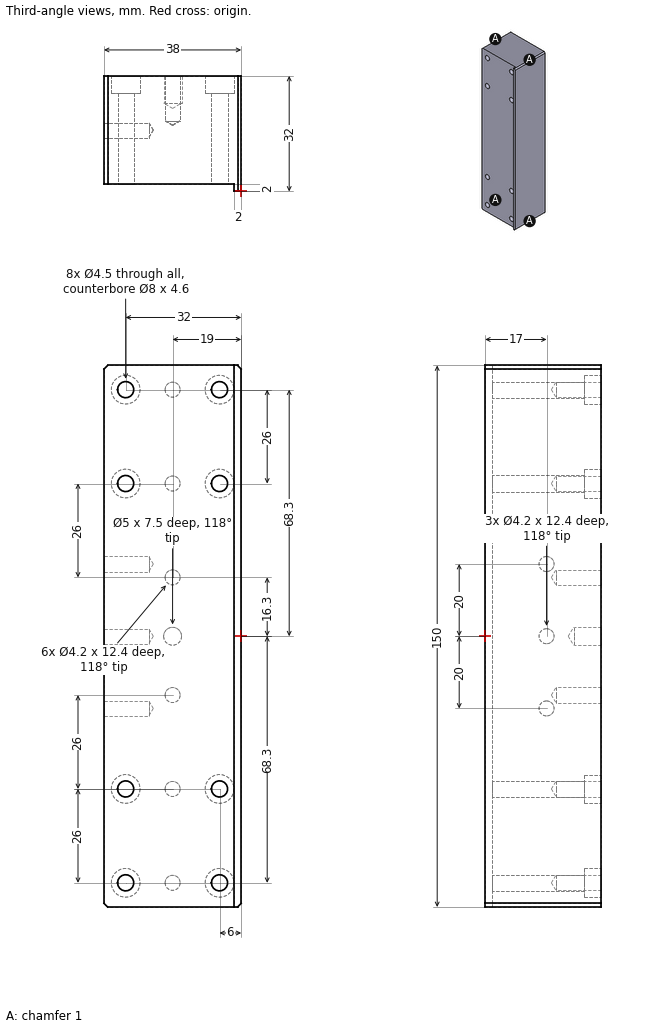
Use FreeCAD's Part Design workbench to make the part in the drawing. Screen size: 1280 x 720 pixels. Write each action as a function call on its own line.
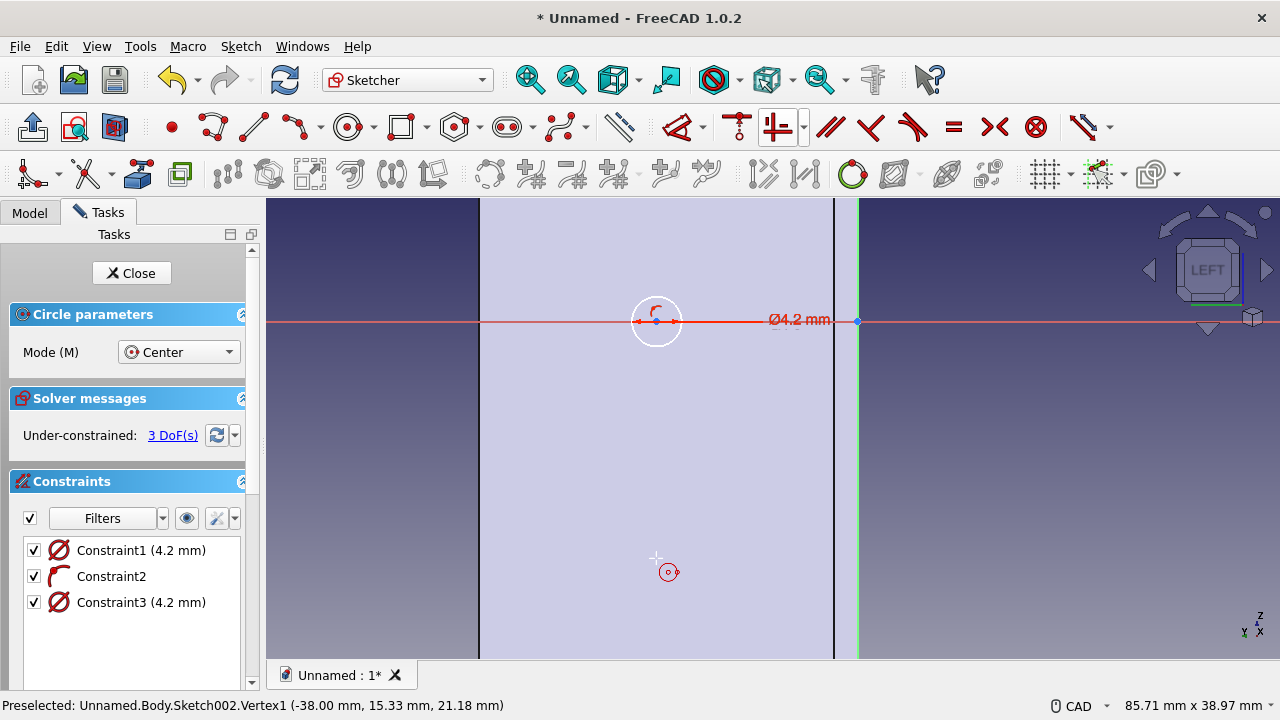
click(656, 558)
move(674, 541)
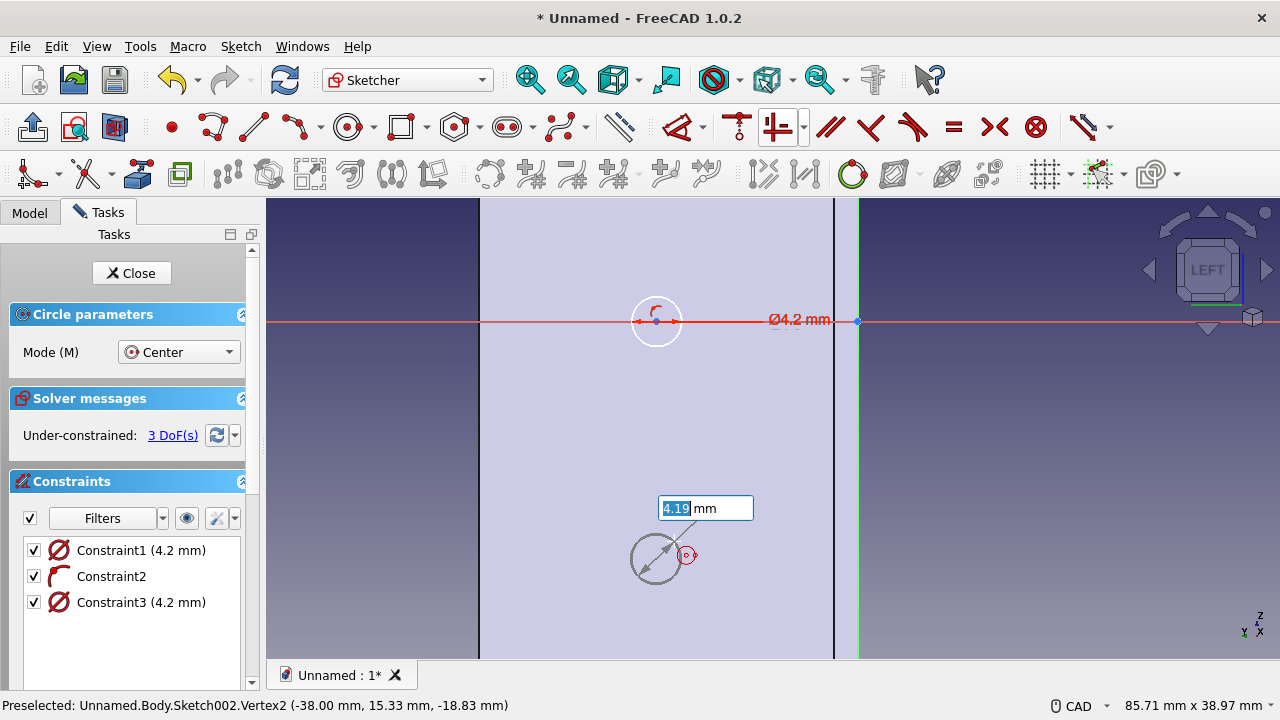
text(4.2)
key(Return)
key(Escape)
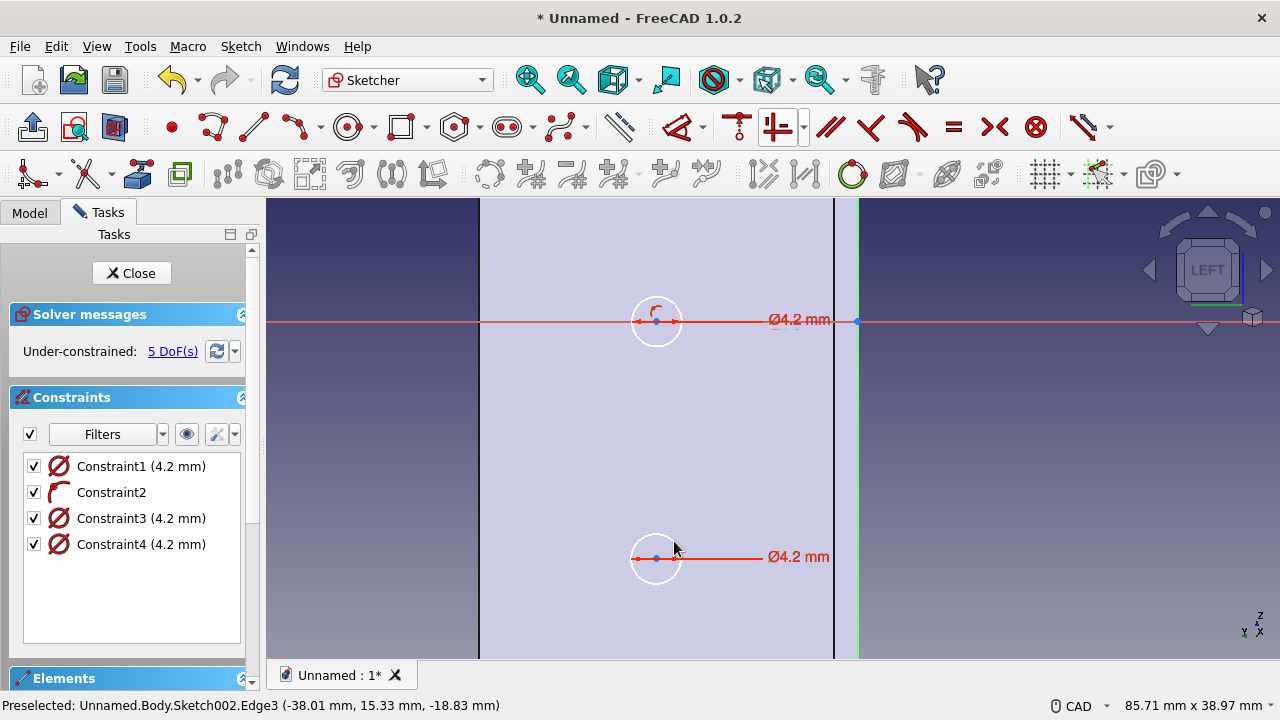
click(676, 128)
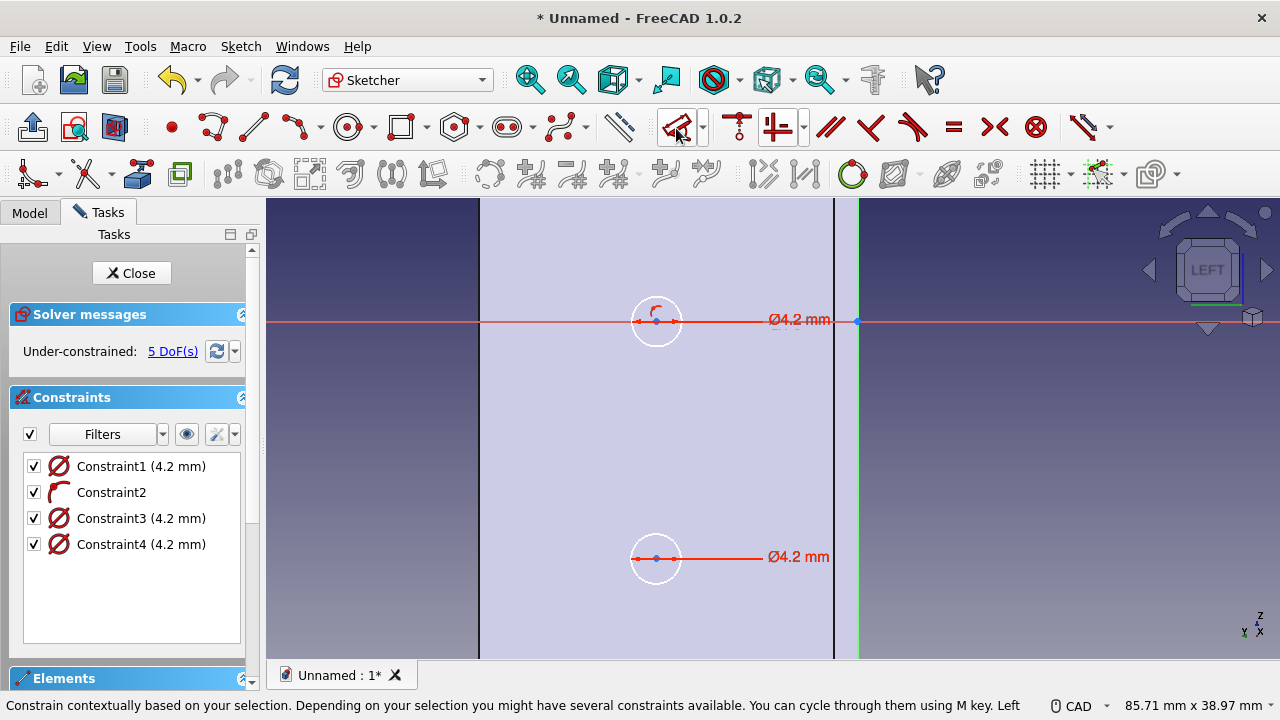
click(657, 322)
click(757, 356)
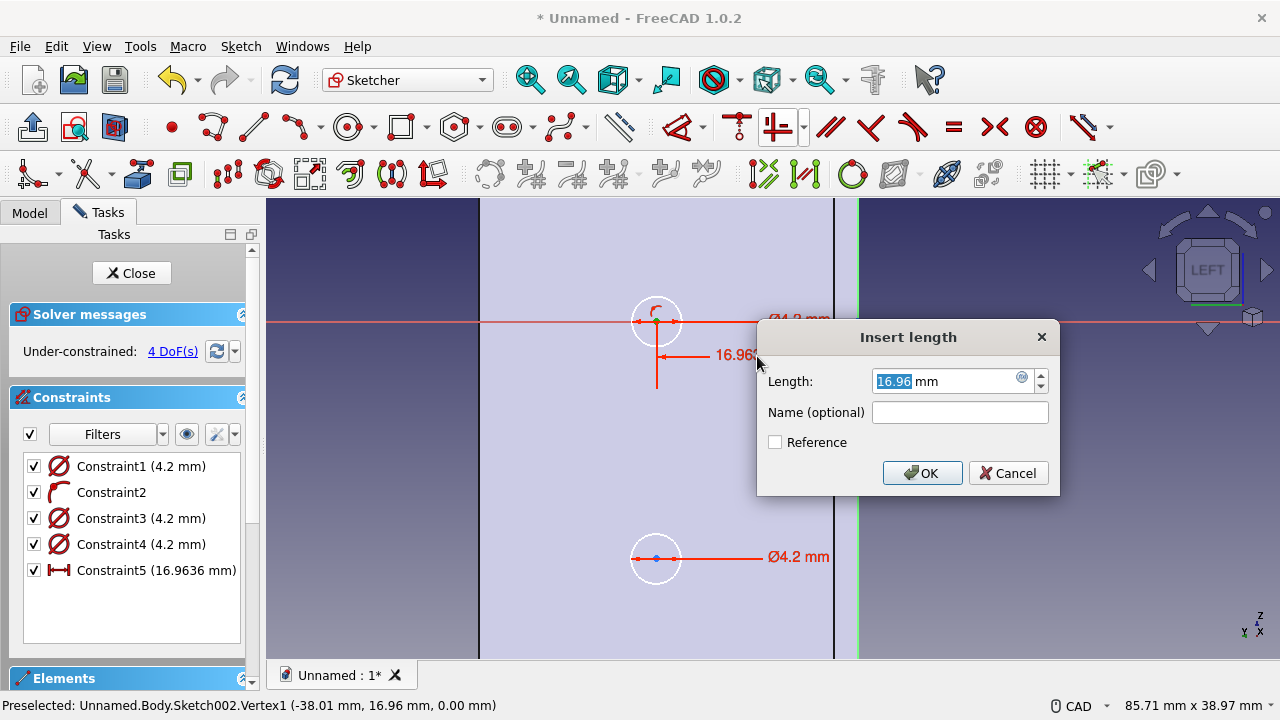
text(17)
key(Return)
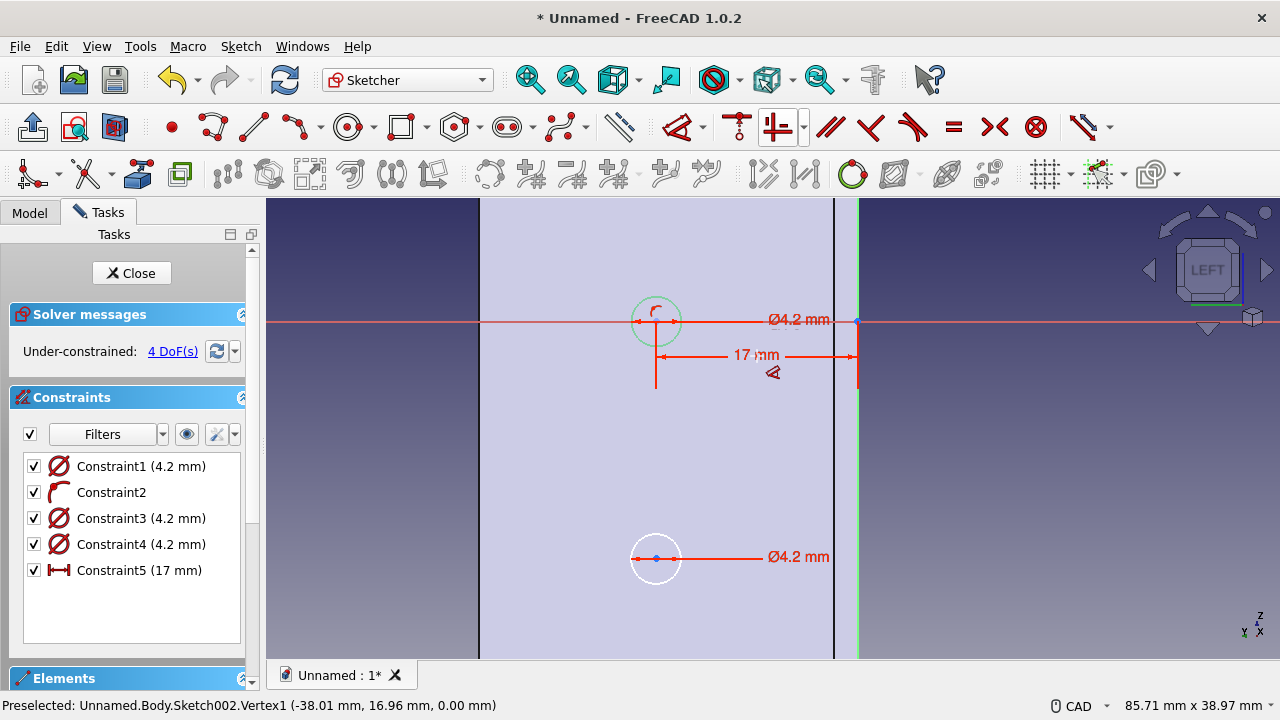
scroll(656, 558, down, 3)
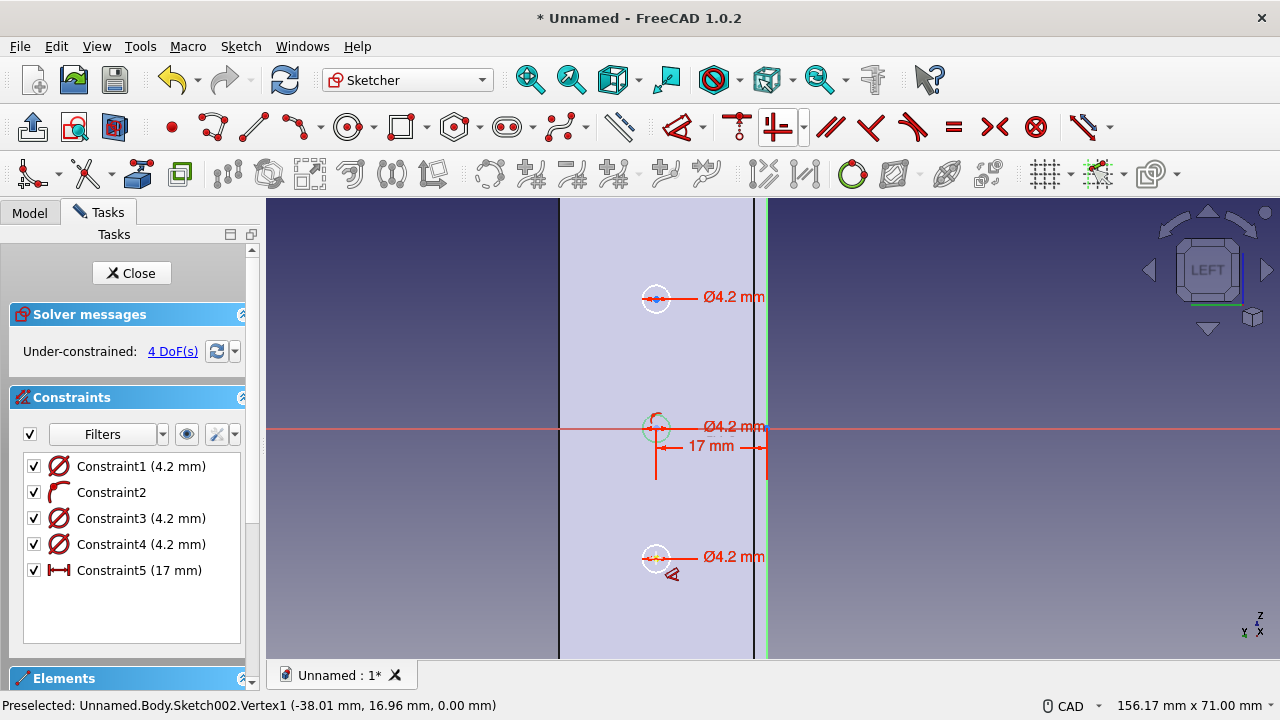
click(656, 299)
click(711, 265)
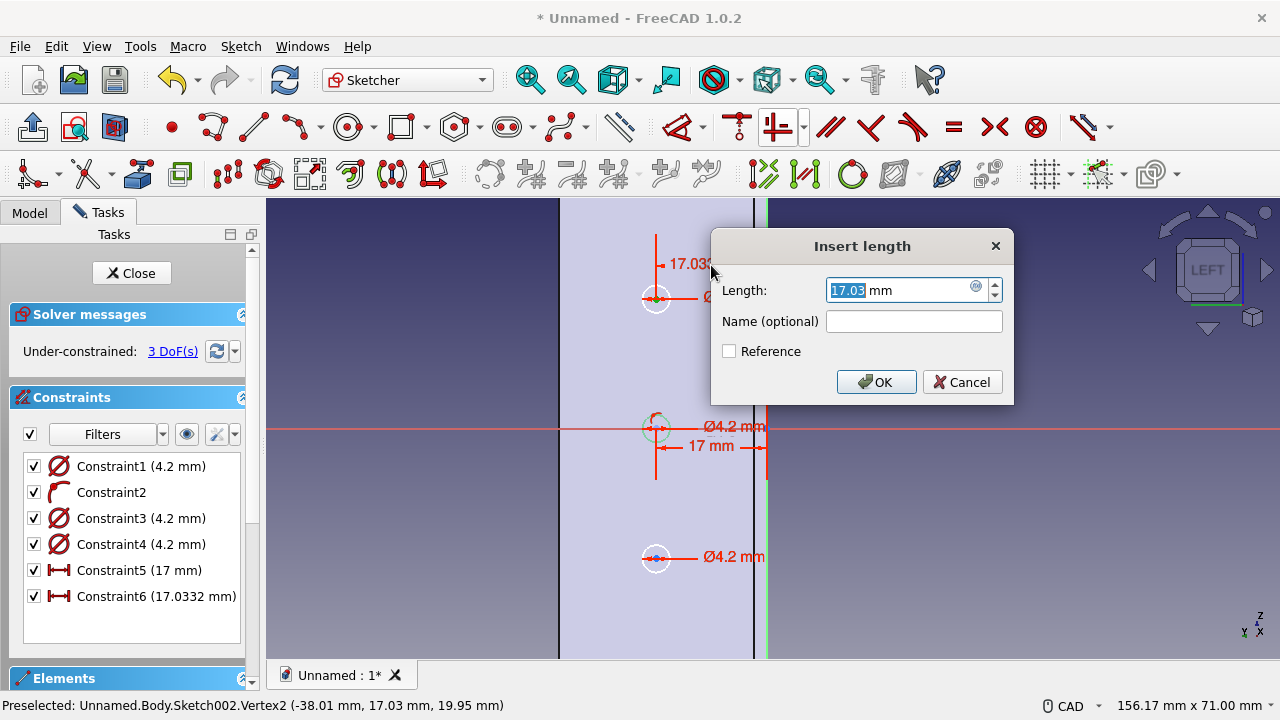
text(17)
key(Return)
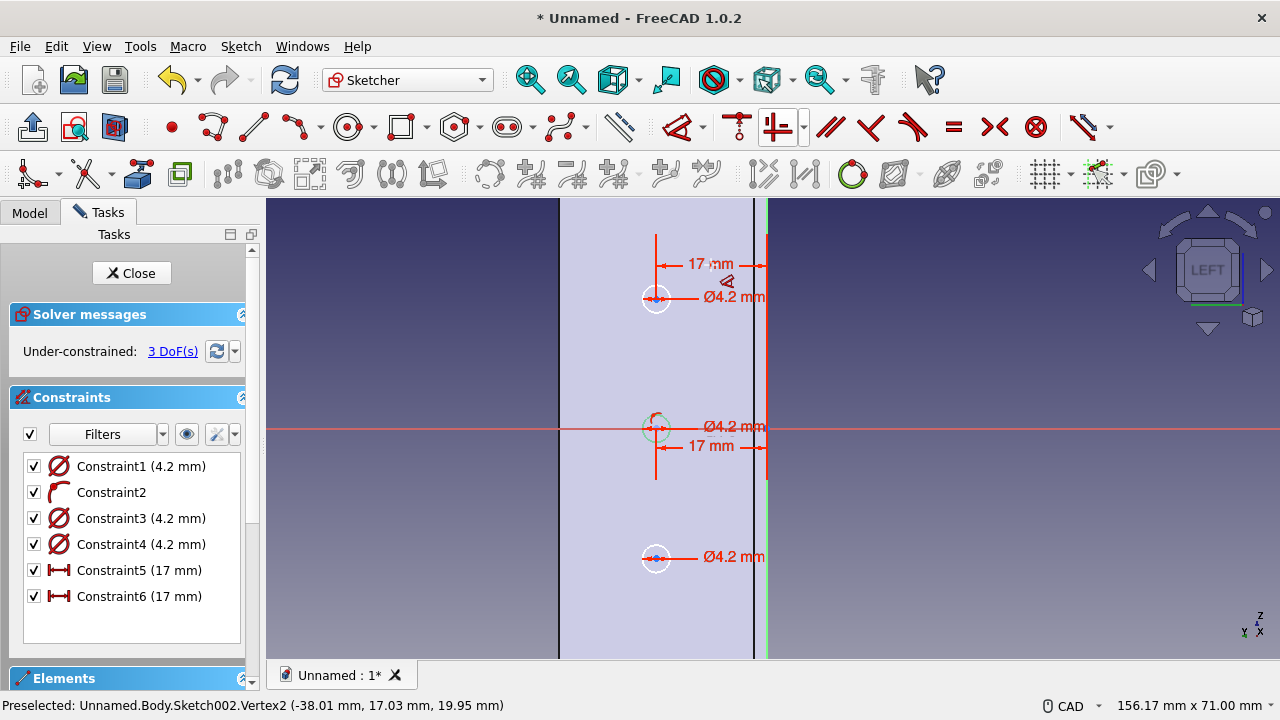
click(656, 299)
click(801, 364)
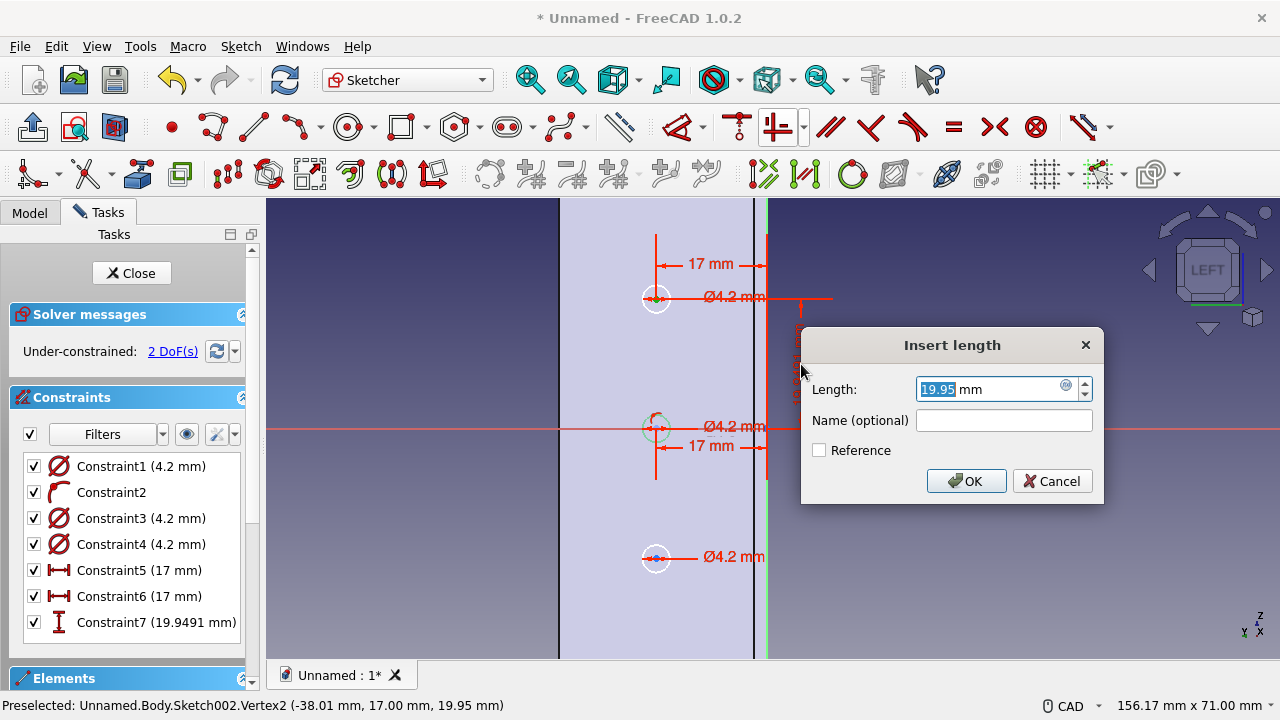
text(20)
key(Return)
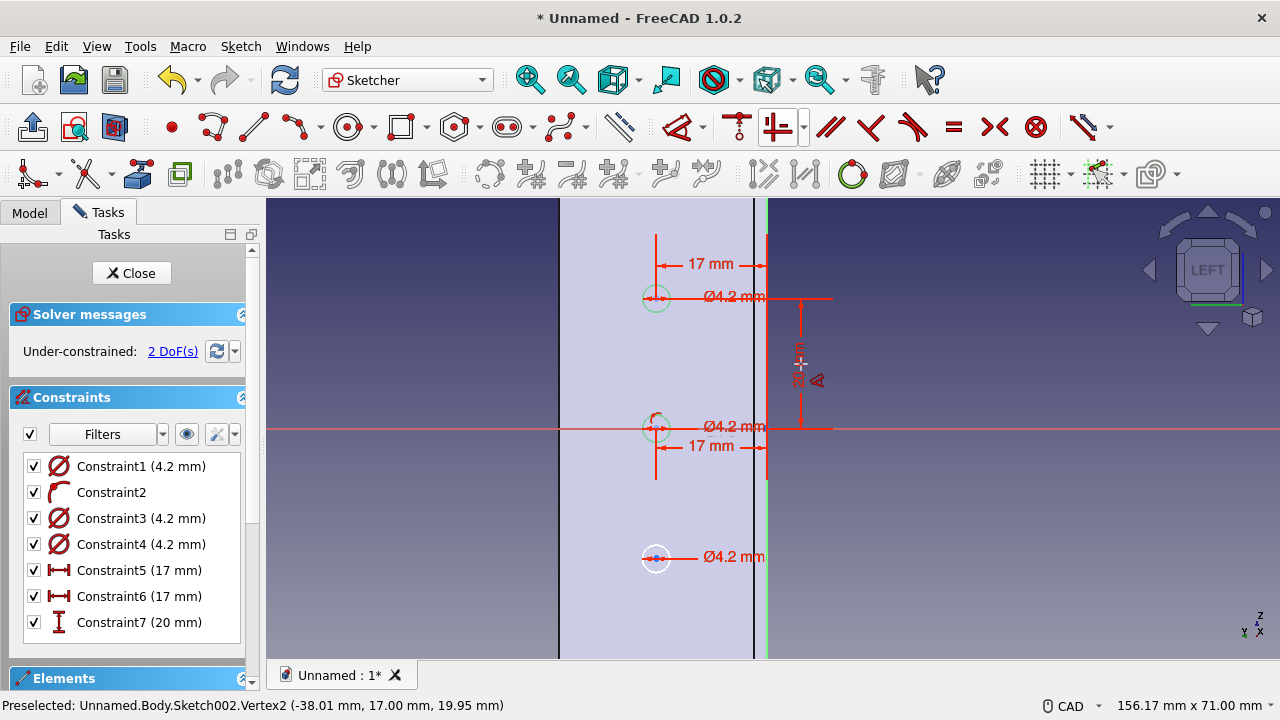
click(656, 559)
click(711, 593)